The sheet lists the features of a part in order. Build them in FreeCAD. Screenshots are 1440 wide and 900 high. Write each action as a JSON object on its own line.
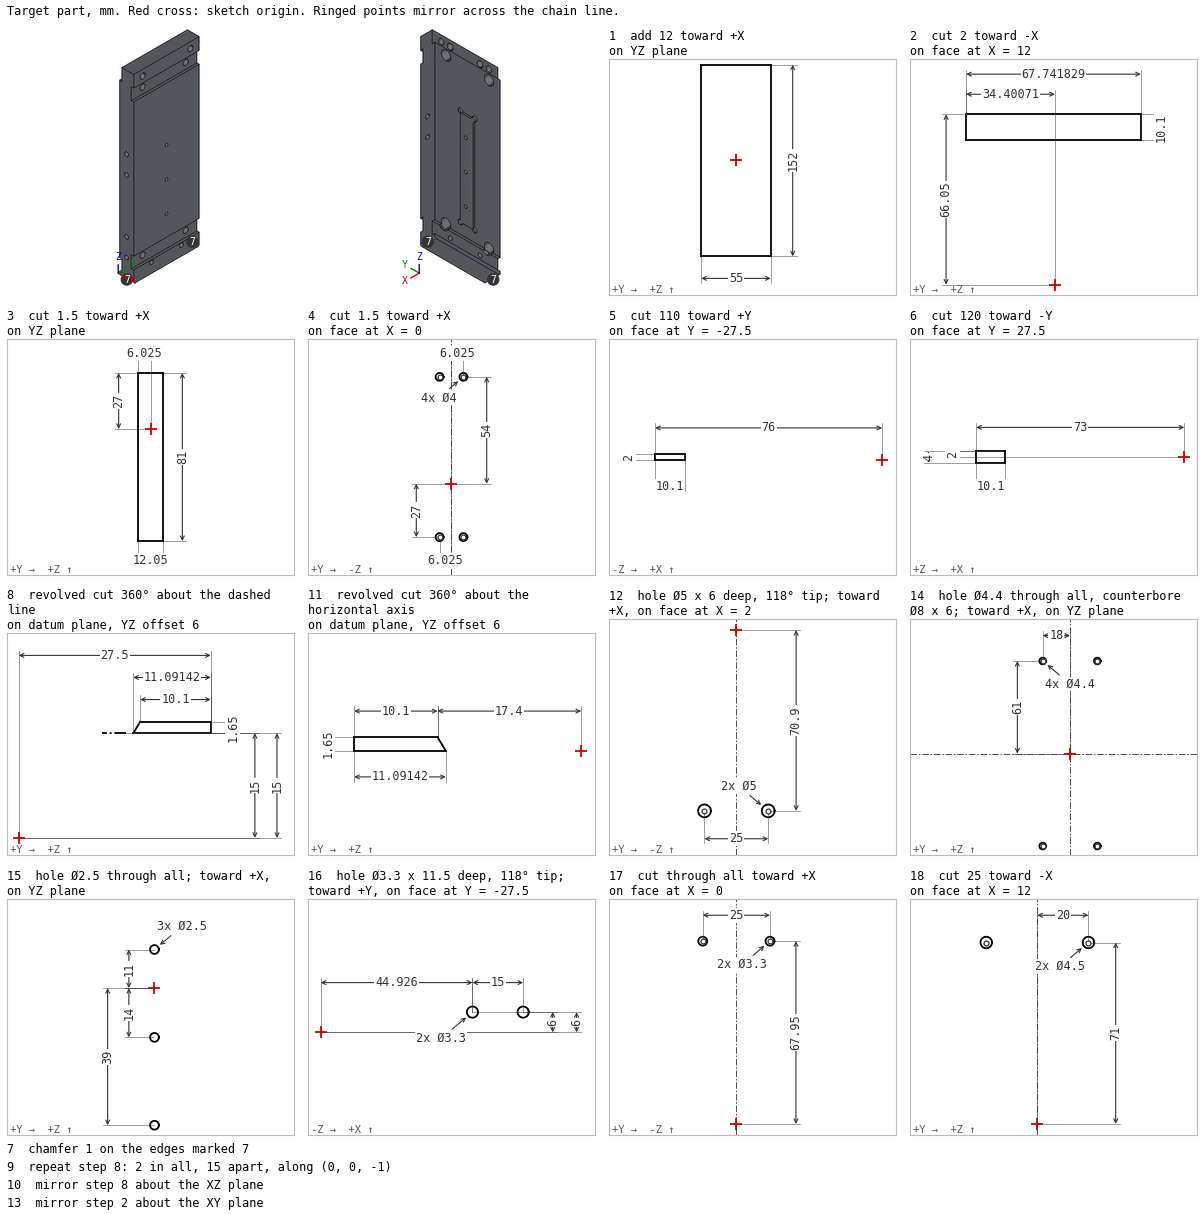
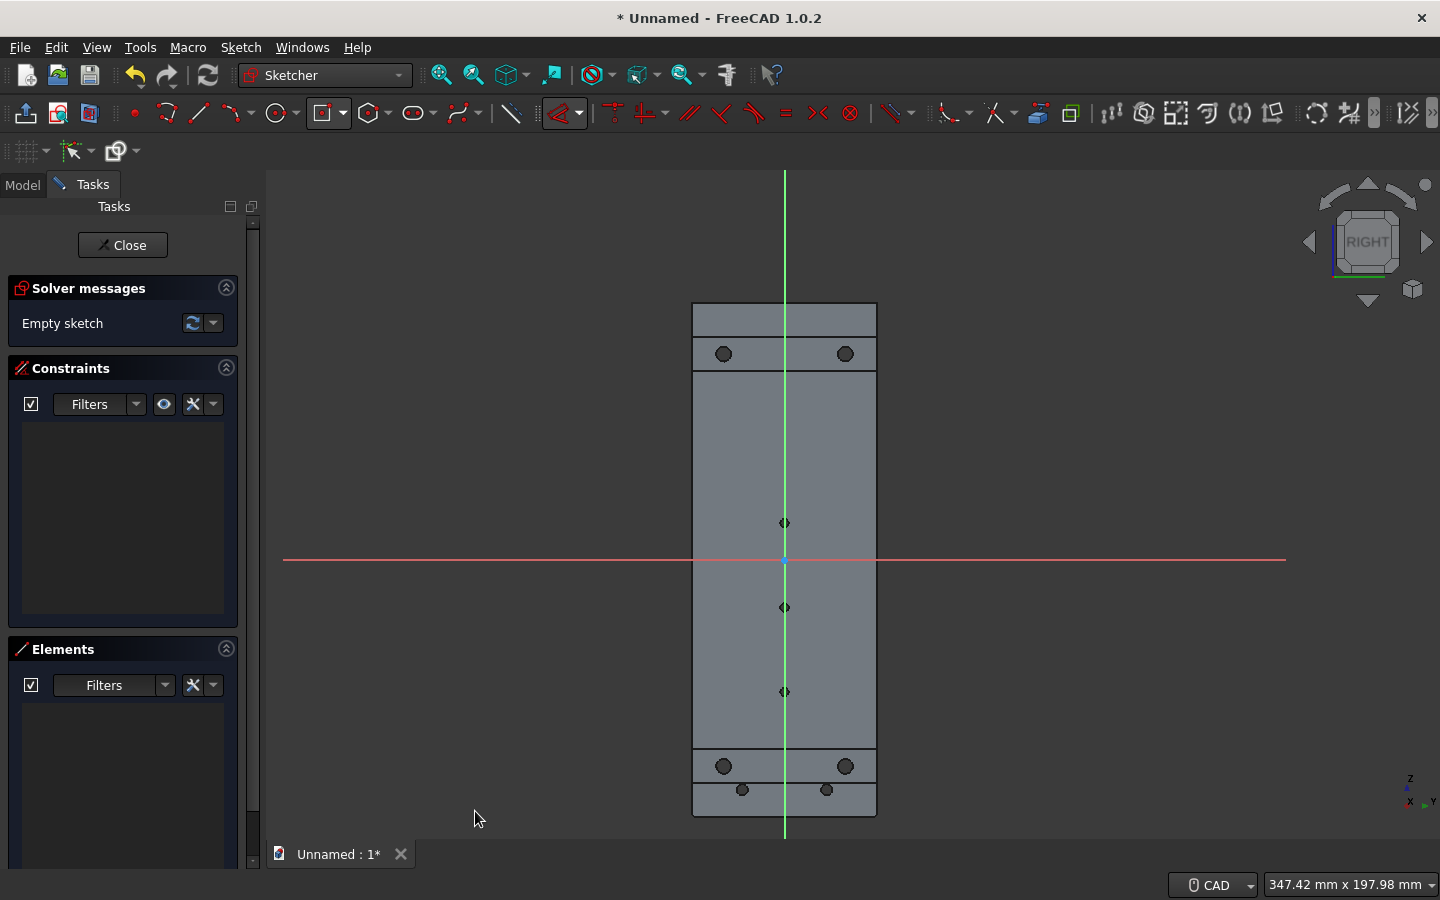
{"action": "scroll", "coordinate": [785, 354], "scroll_direction": "up", "scroll_amount": 3}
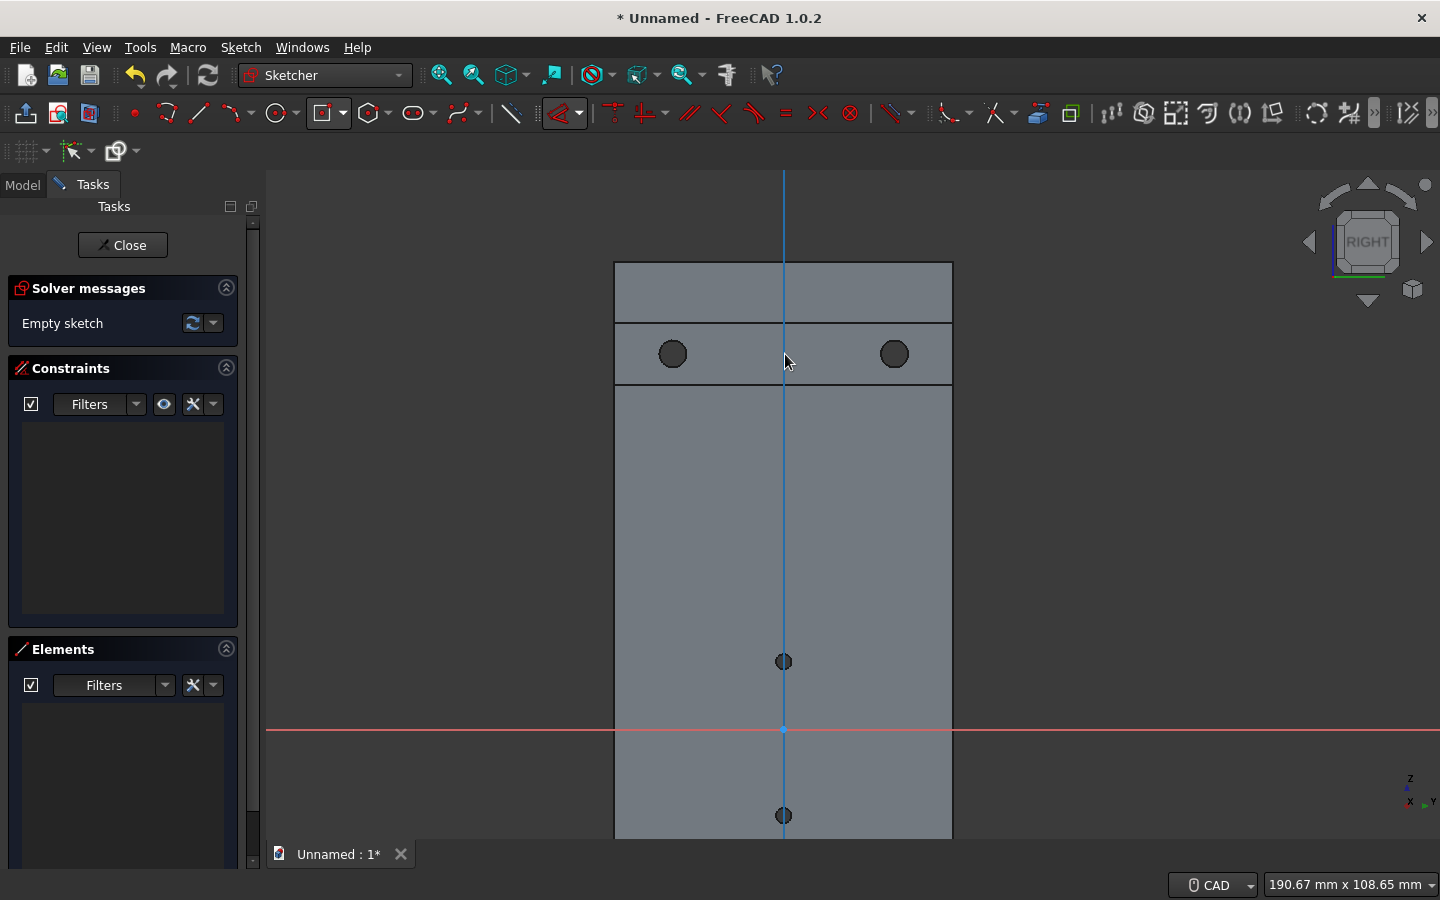
{"action": "left_click", "coordinate": [276, 114]}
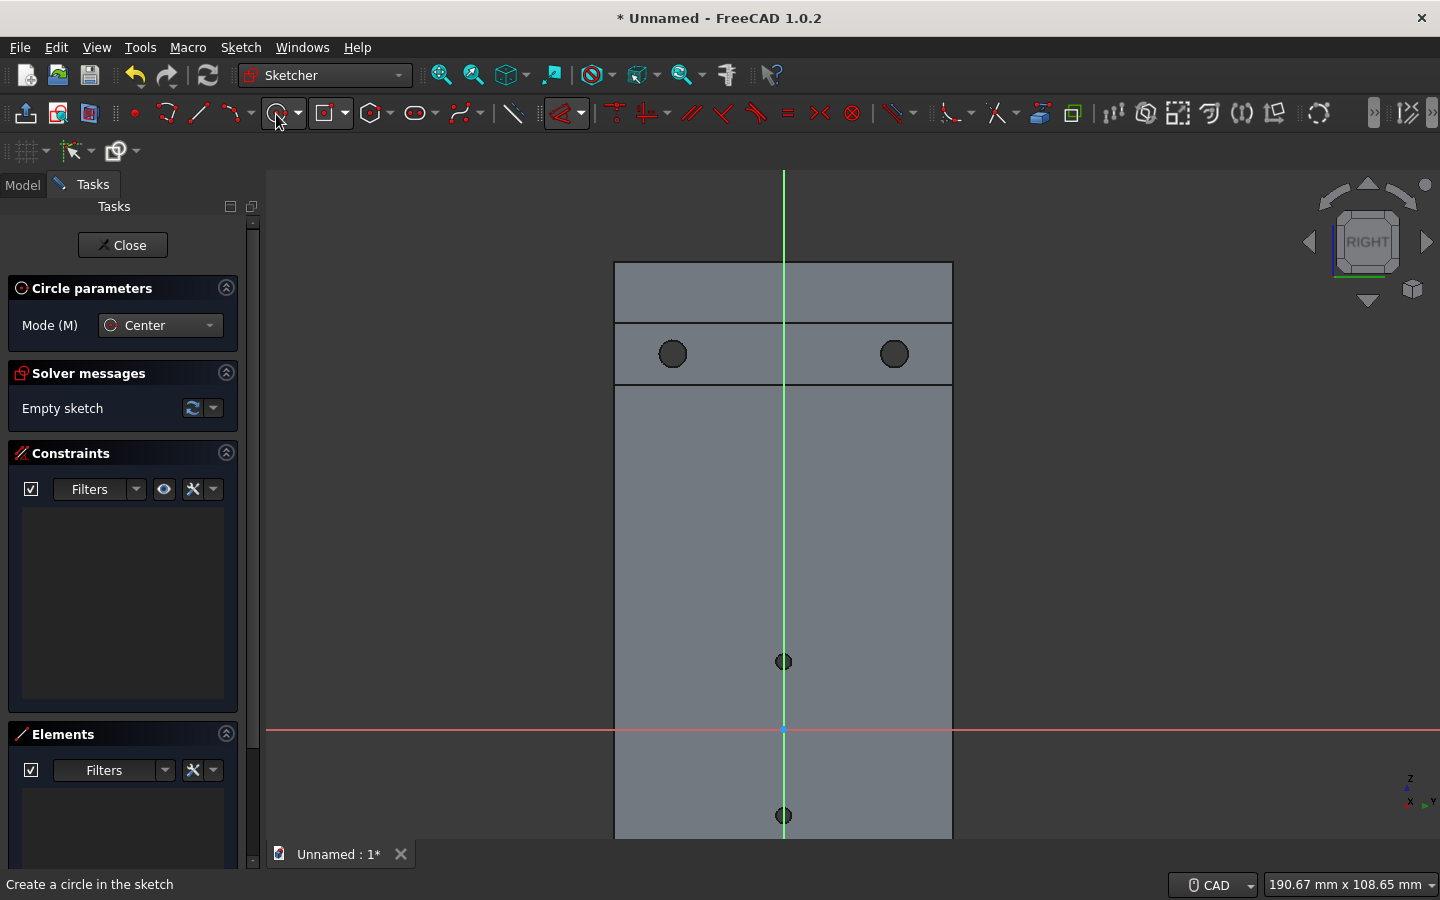
{"action": "scroll", "coordinate": [907, 292], "scroll_direction": "up", "scroll_amount": 3}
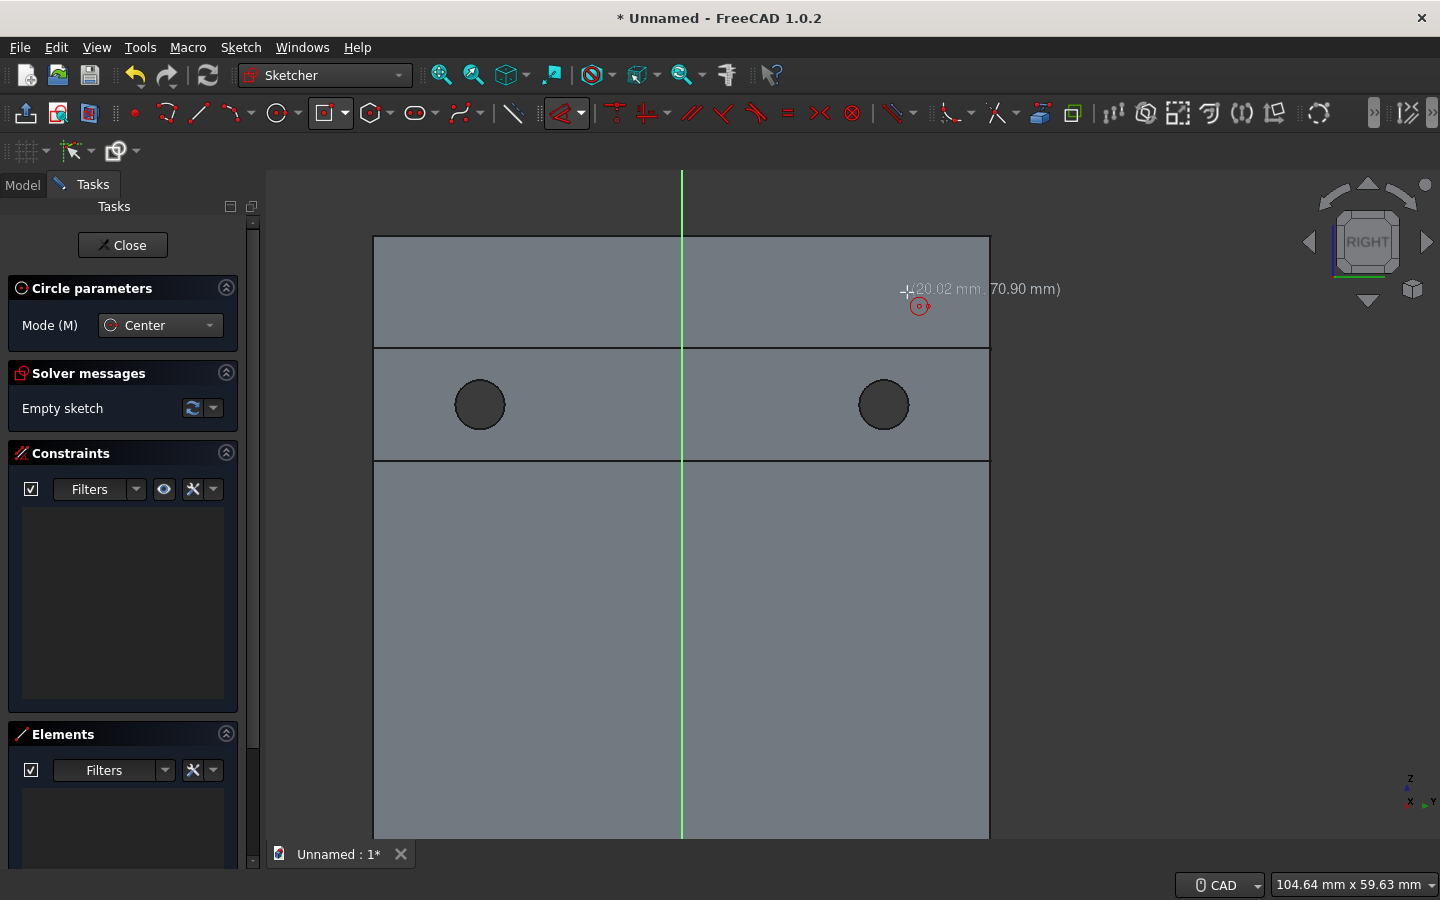
{"action": "left_click", "coordinate": [906, 293]}
{"action": "mouse_move", "coordinate": [924, 275]}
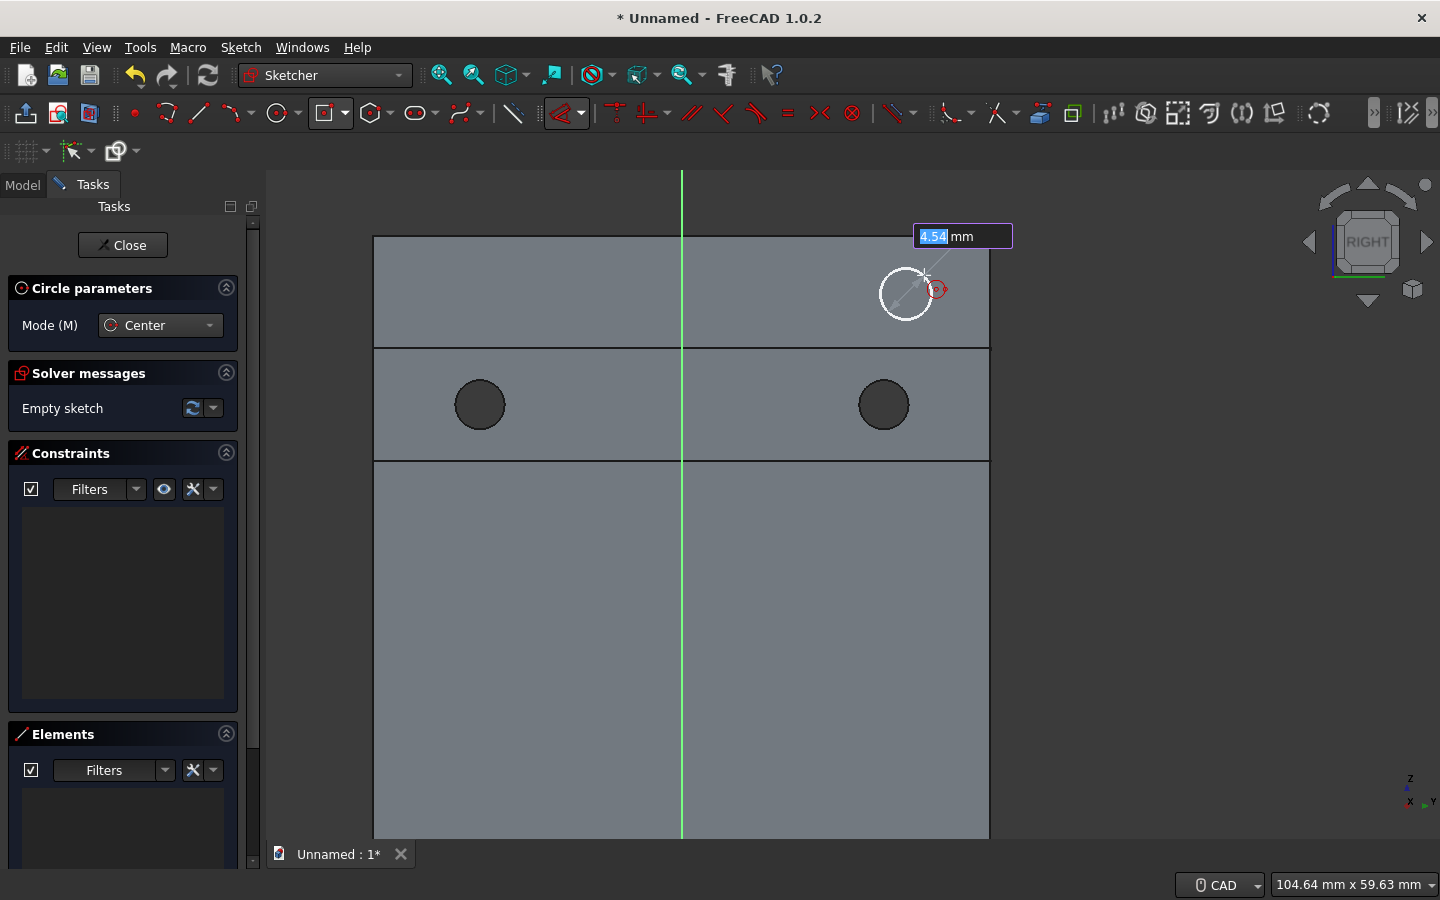
{"action": "type", "text": "4.5"}
{"action": "key", "text": "Return"}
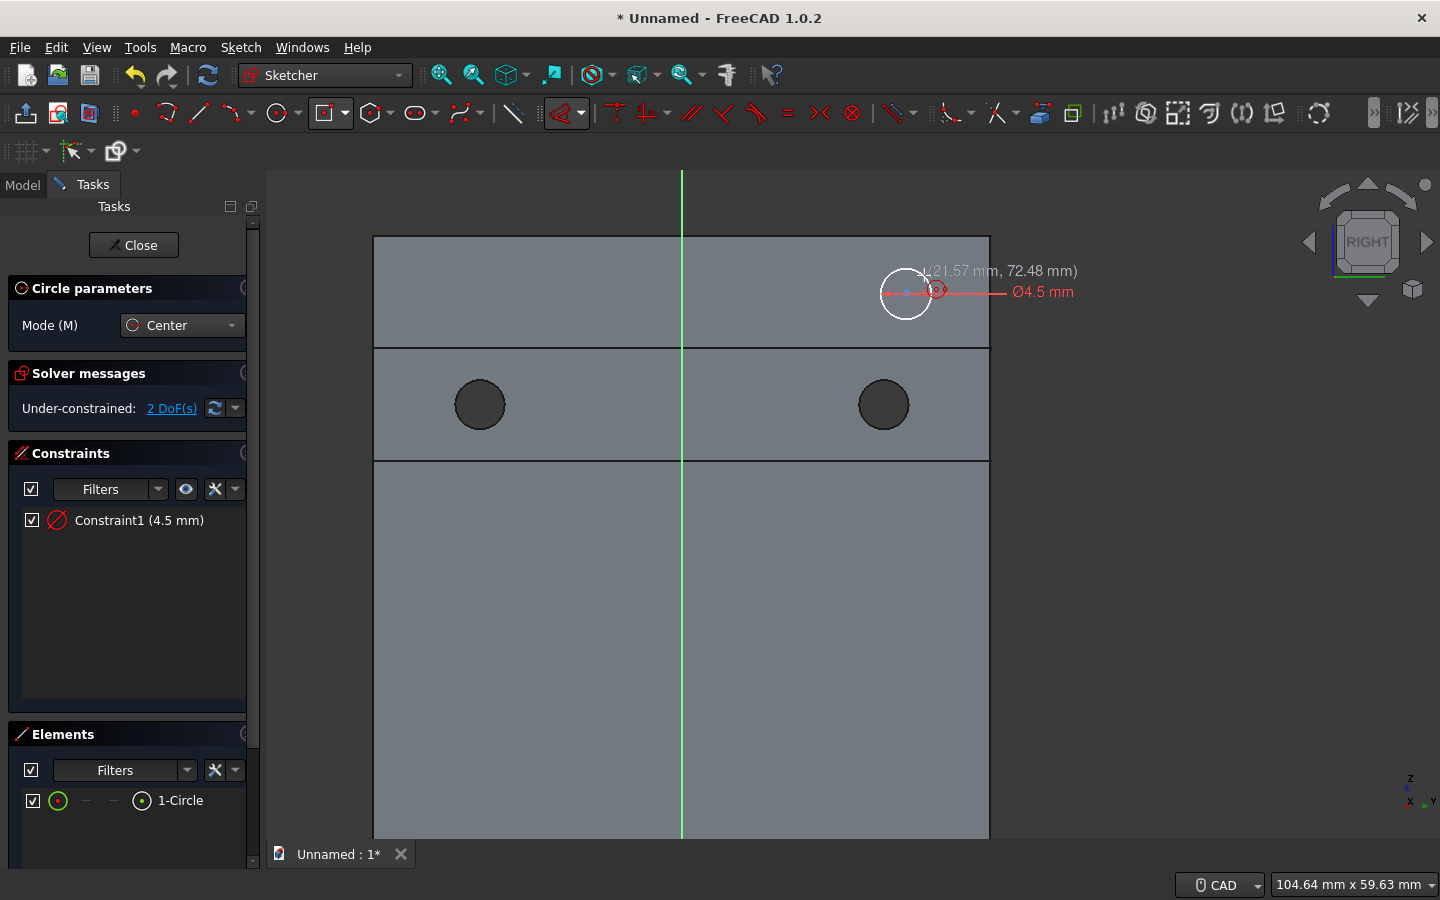
{"action": "left_click", "coordinate": [458, 293]}
{"action": "mouse_move", "coordinate": [475, 275]}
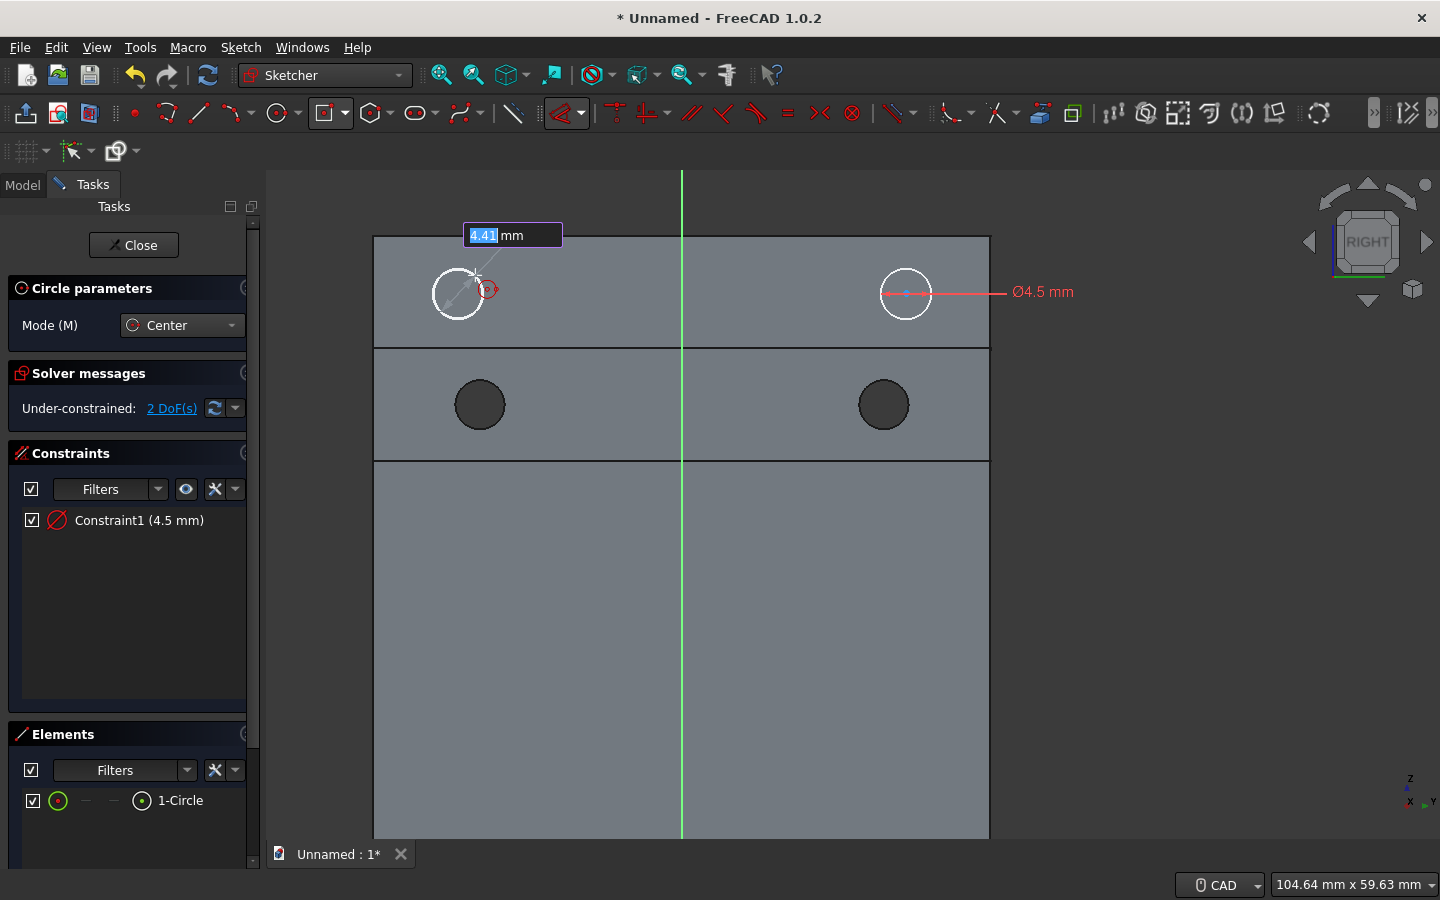
{"action": "type", "text": "4.5"}
{"action": "key", "text": "Return"}
{"action": "key", "text": "Escape"}